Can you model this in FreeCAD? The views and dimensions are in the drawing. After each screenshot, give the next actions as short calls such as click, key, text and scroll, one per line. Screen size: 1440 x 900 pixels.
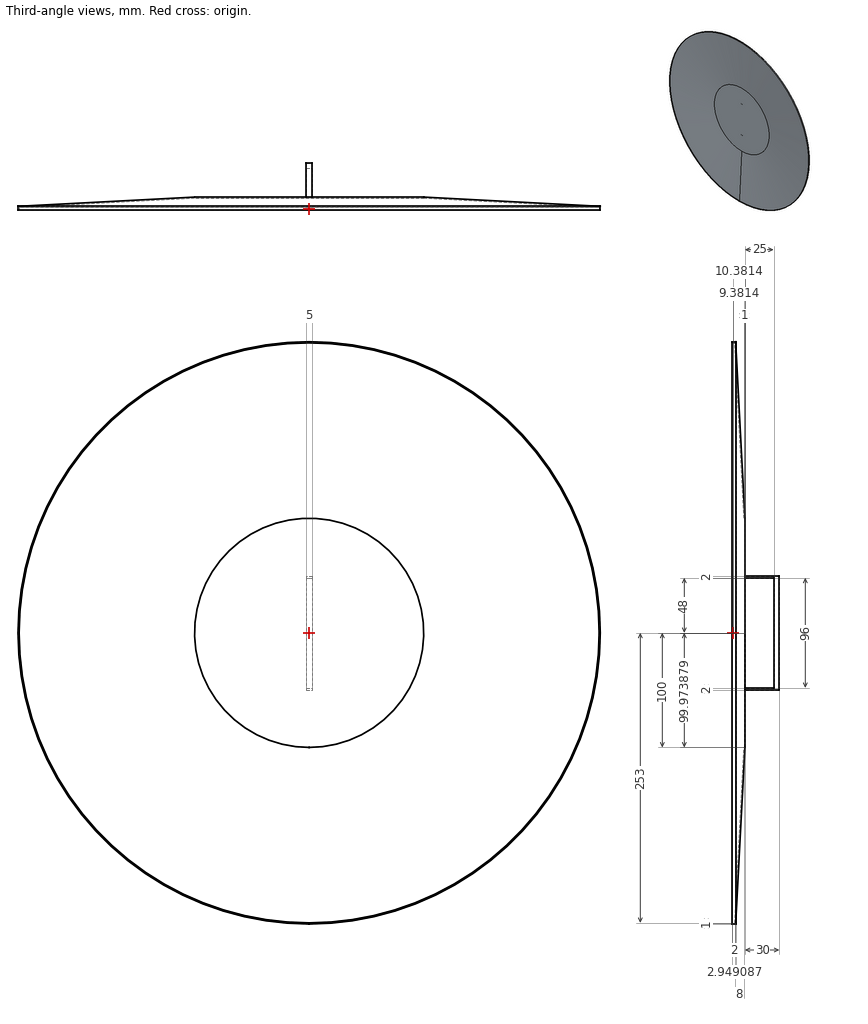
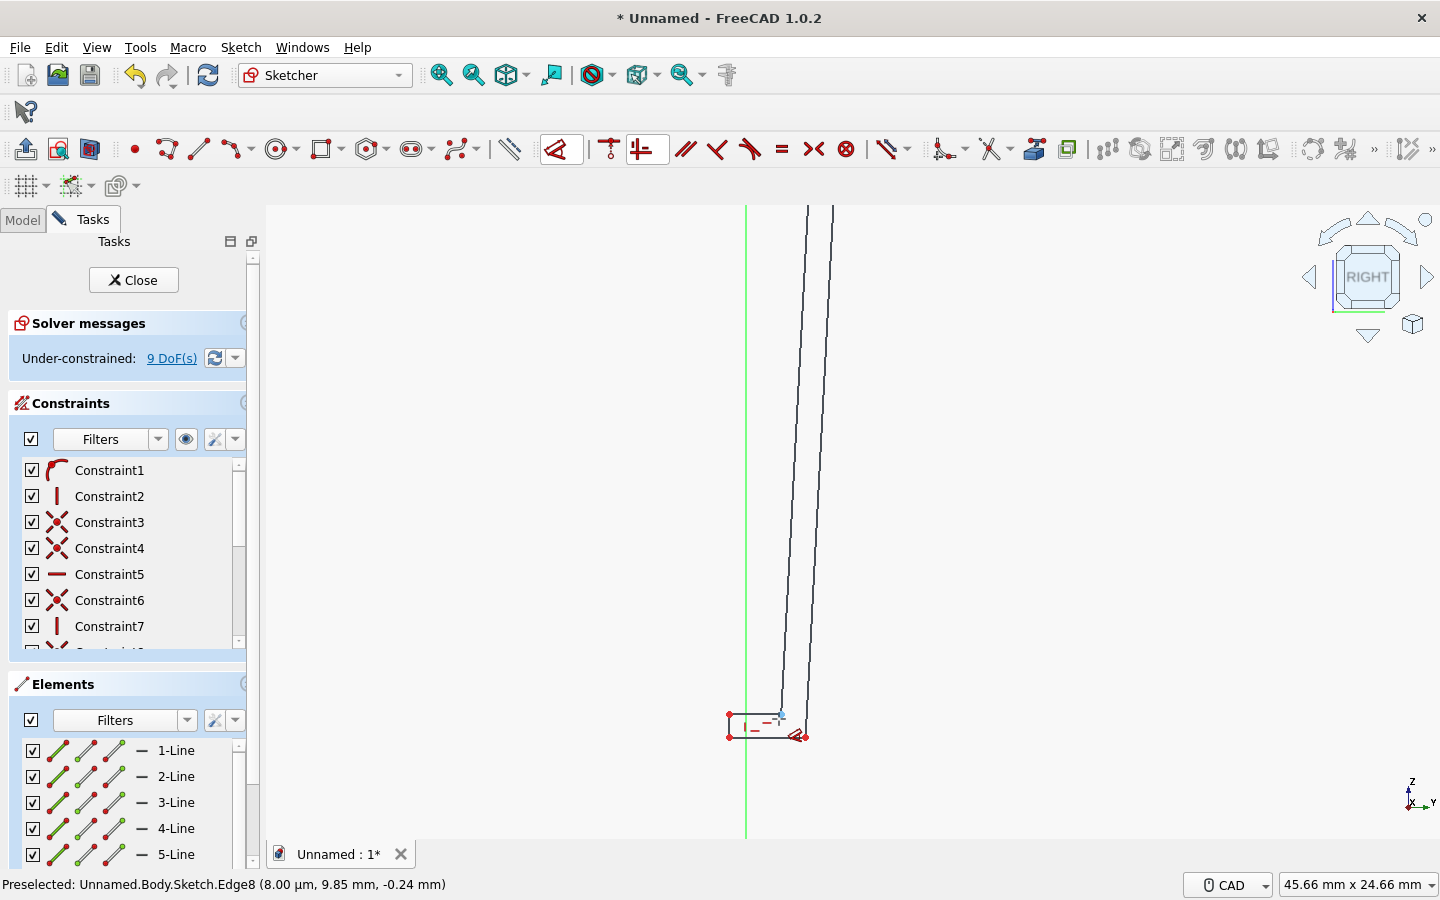
click(766, 714)
click(767, 680)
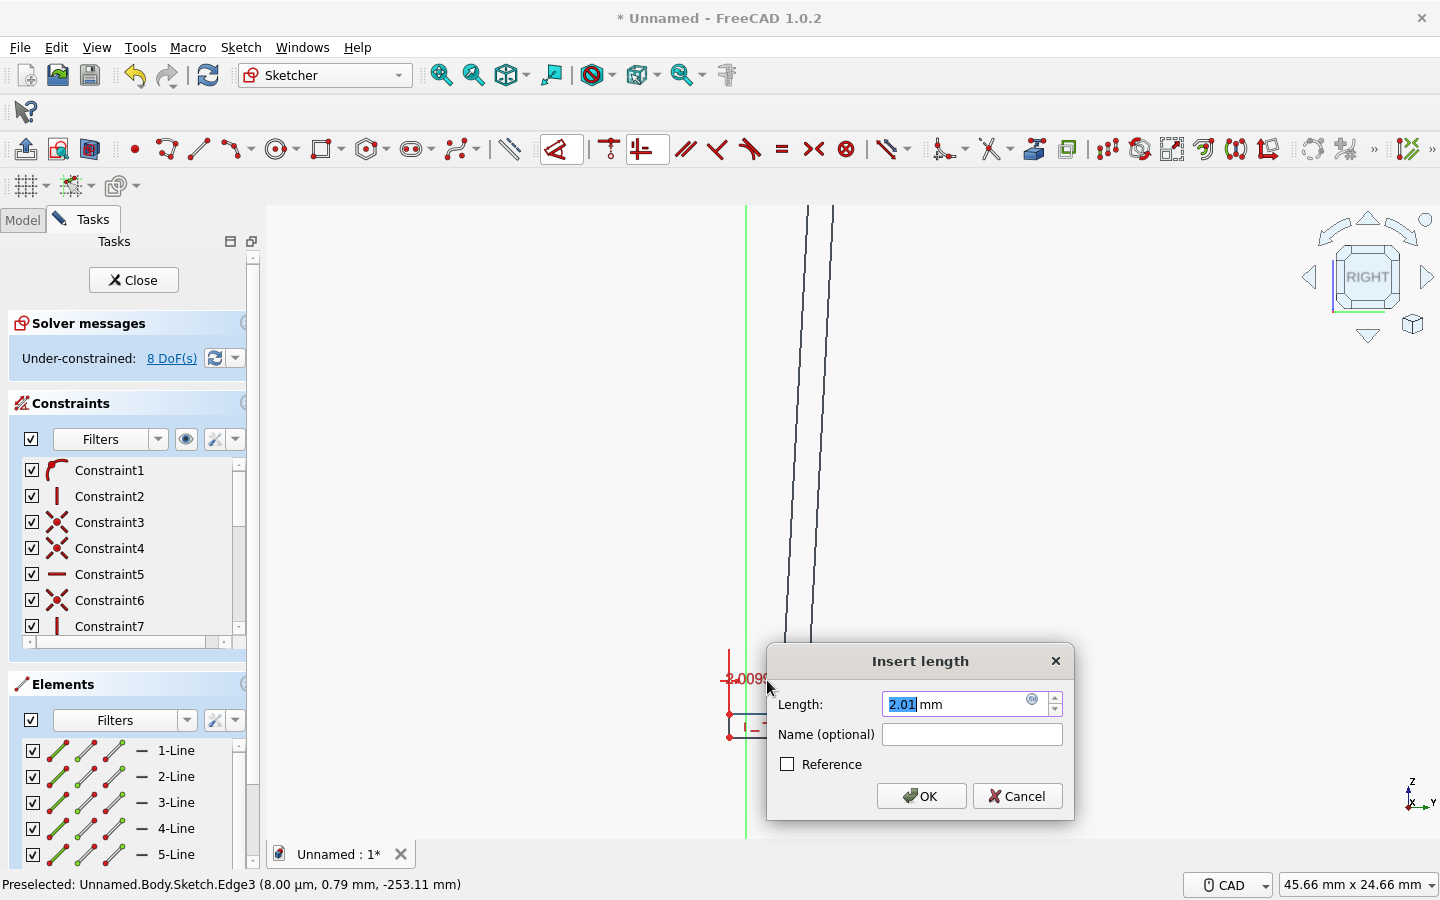
text(2)
key(Return)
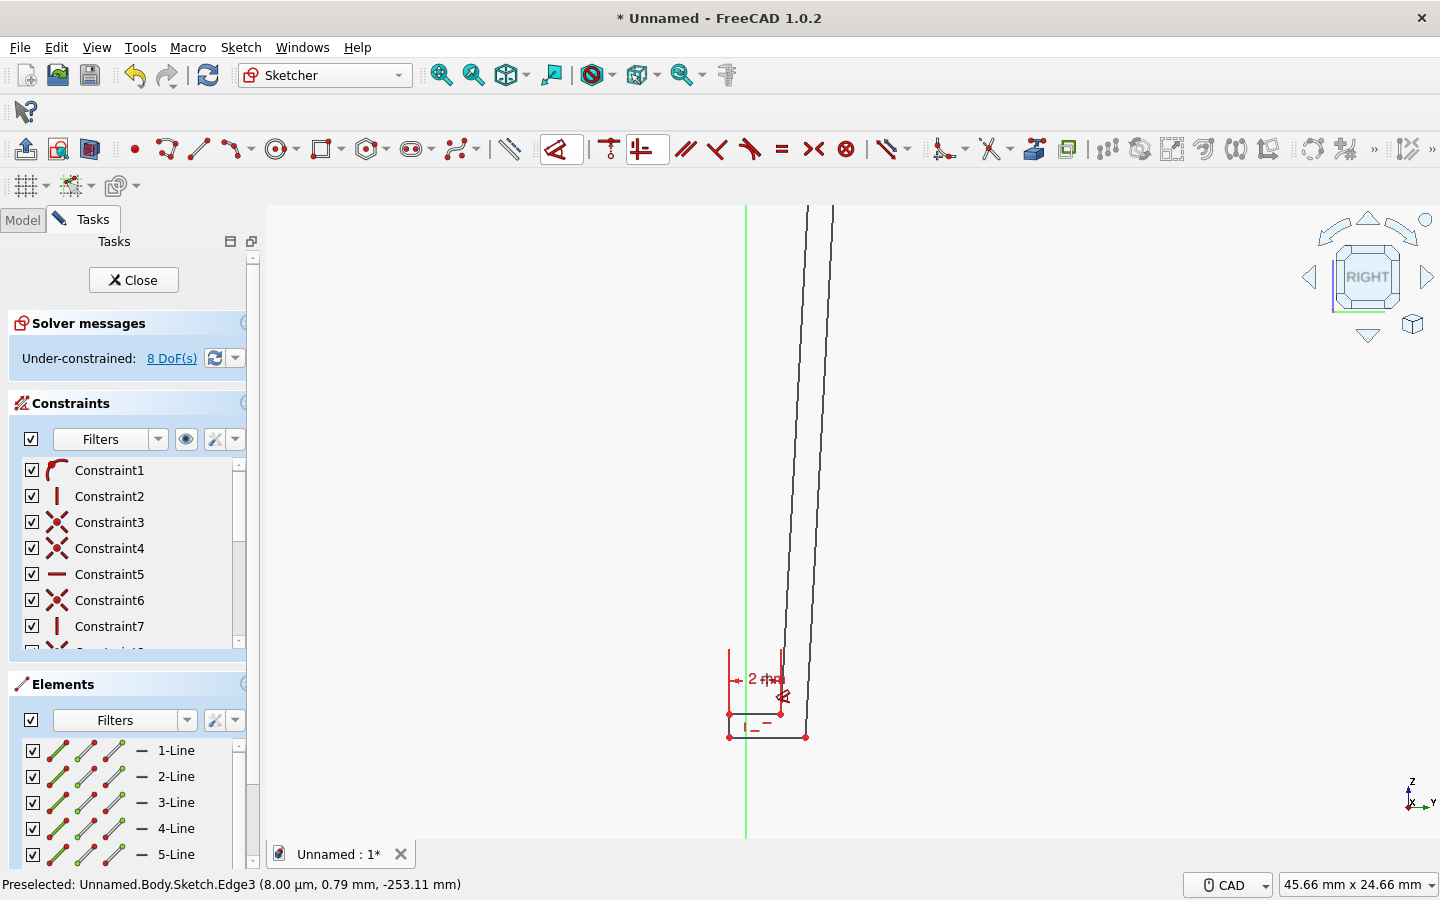
scroll(729, 724, up, 3)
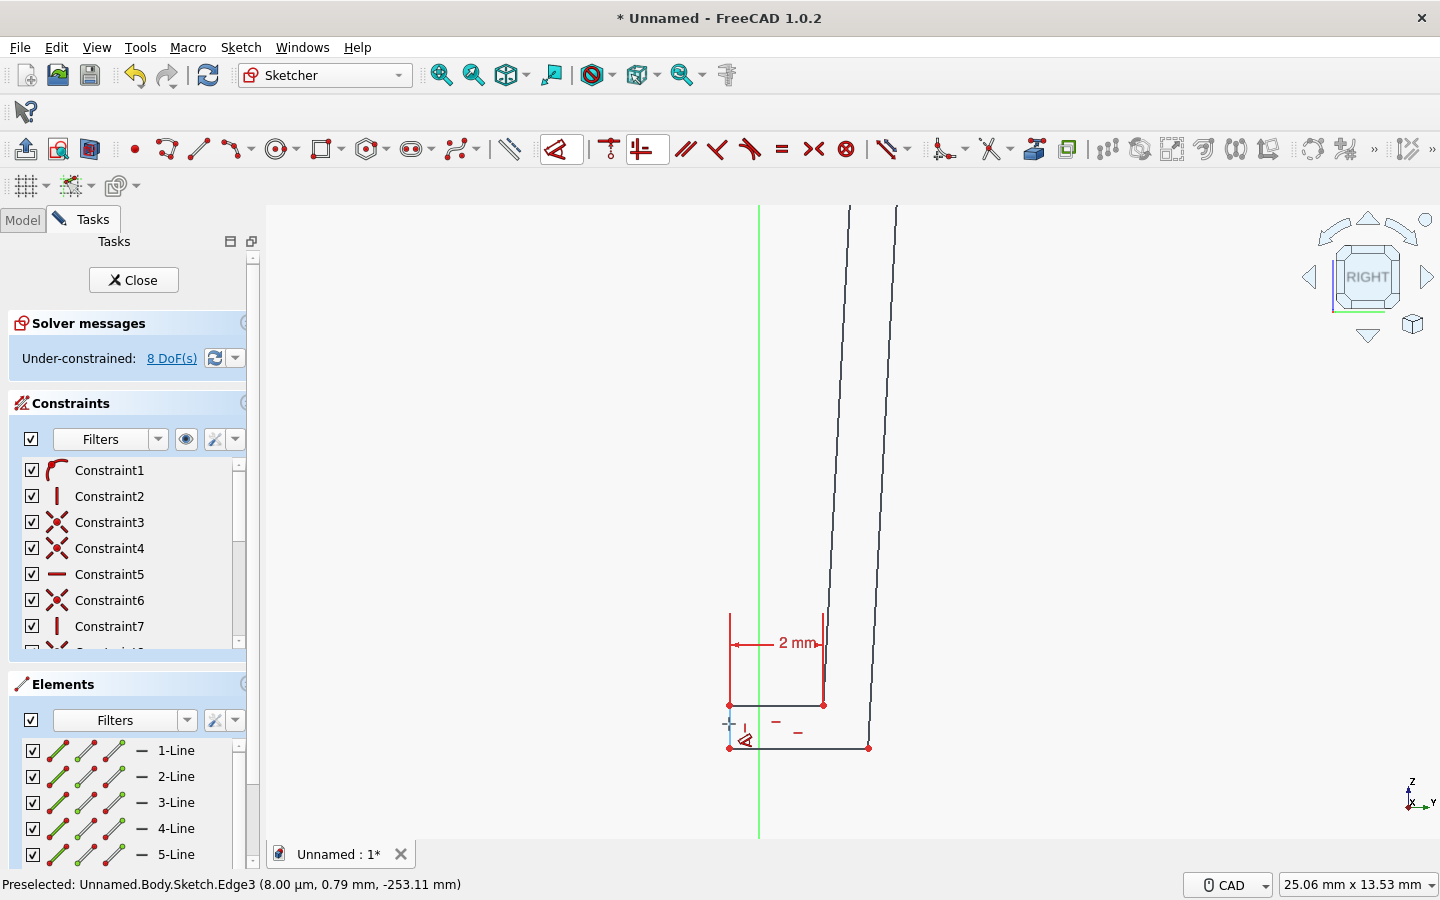
click(730, 723)
click(696, 727)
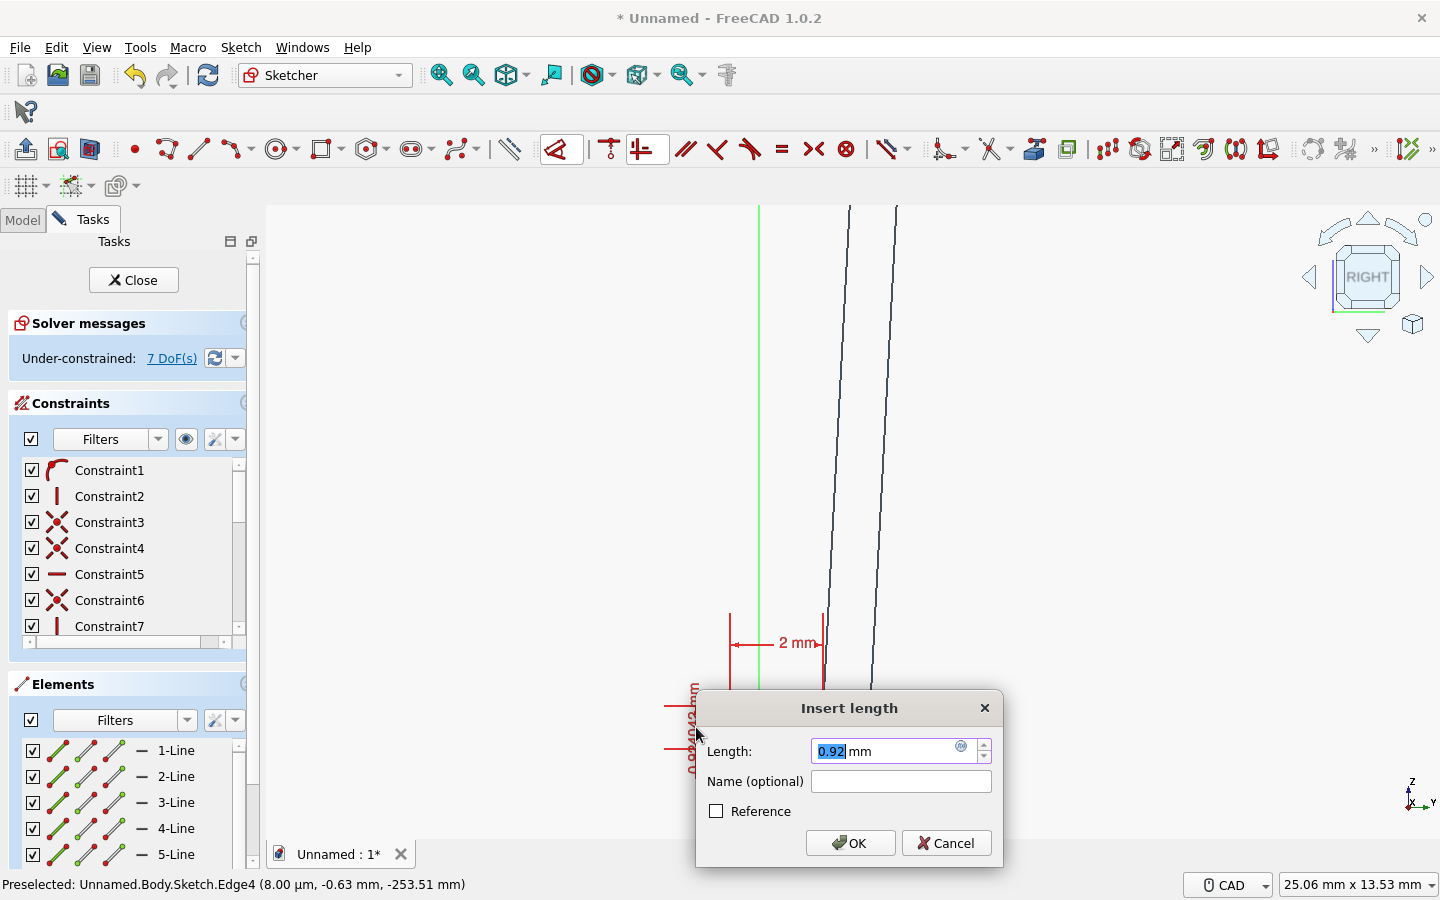
text(1)
key(Return)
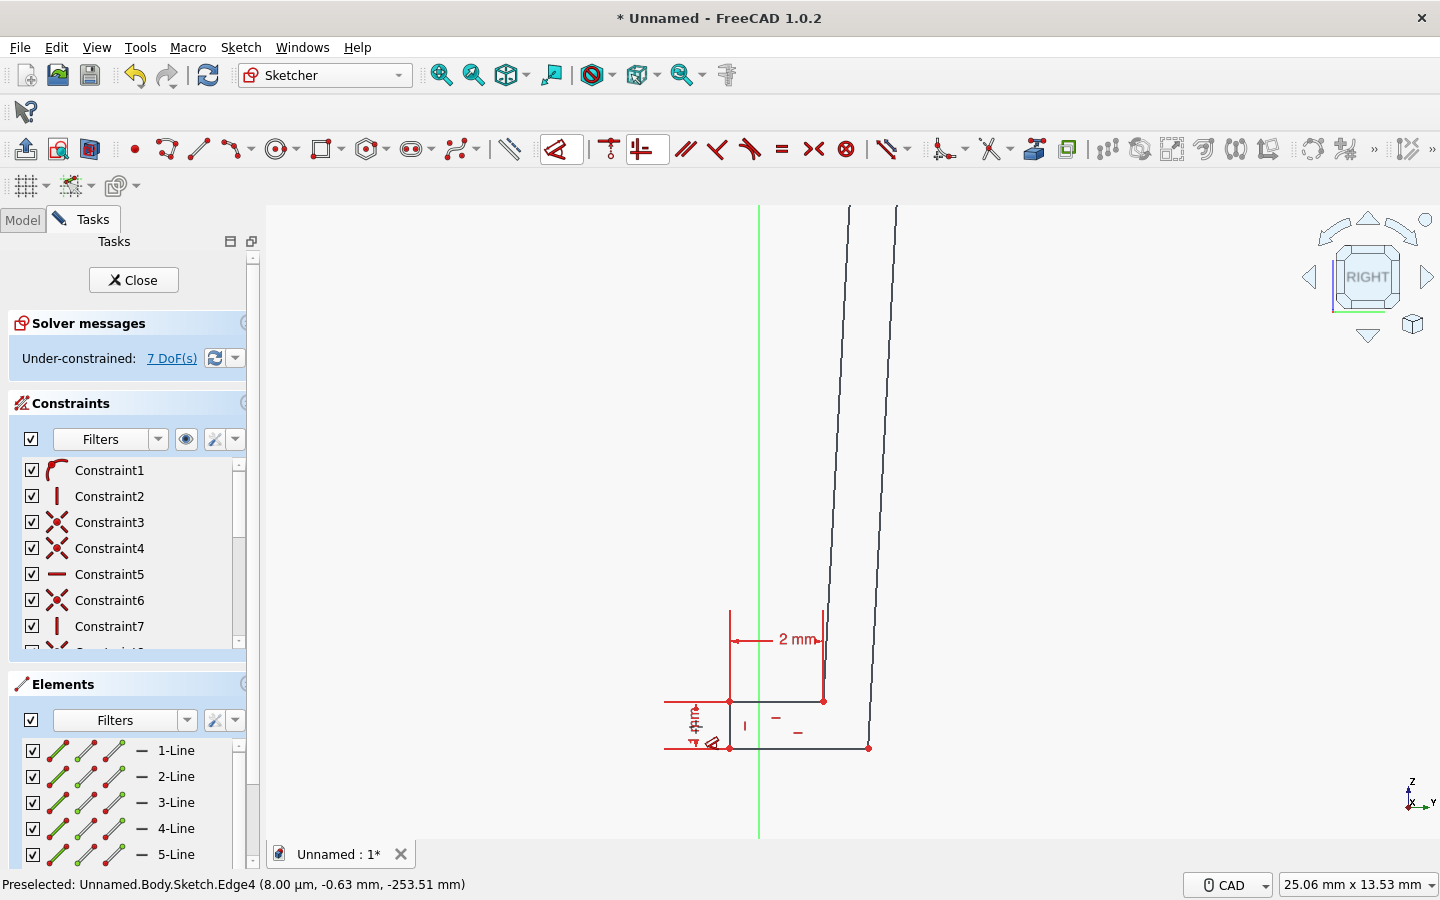
scroll(776, 765, down, 16)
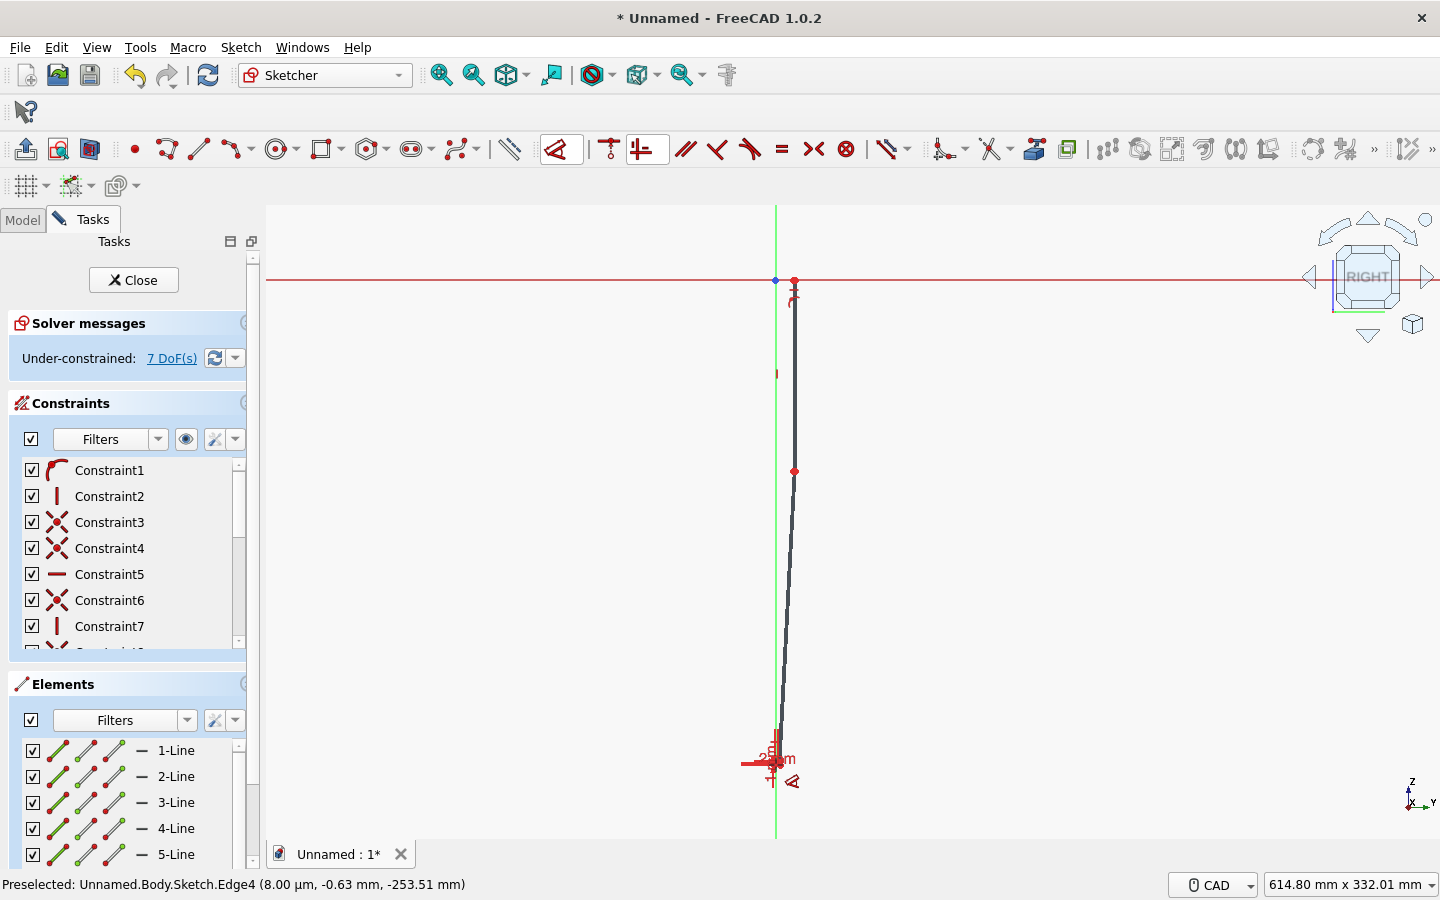
scroll(795, 280, up, 16)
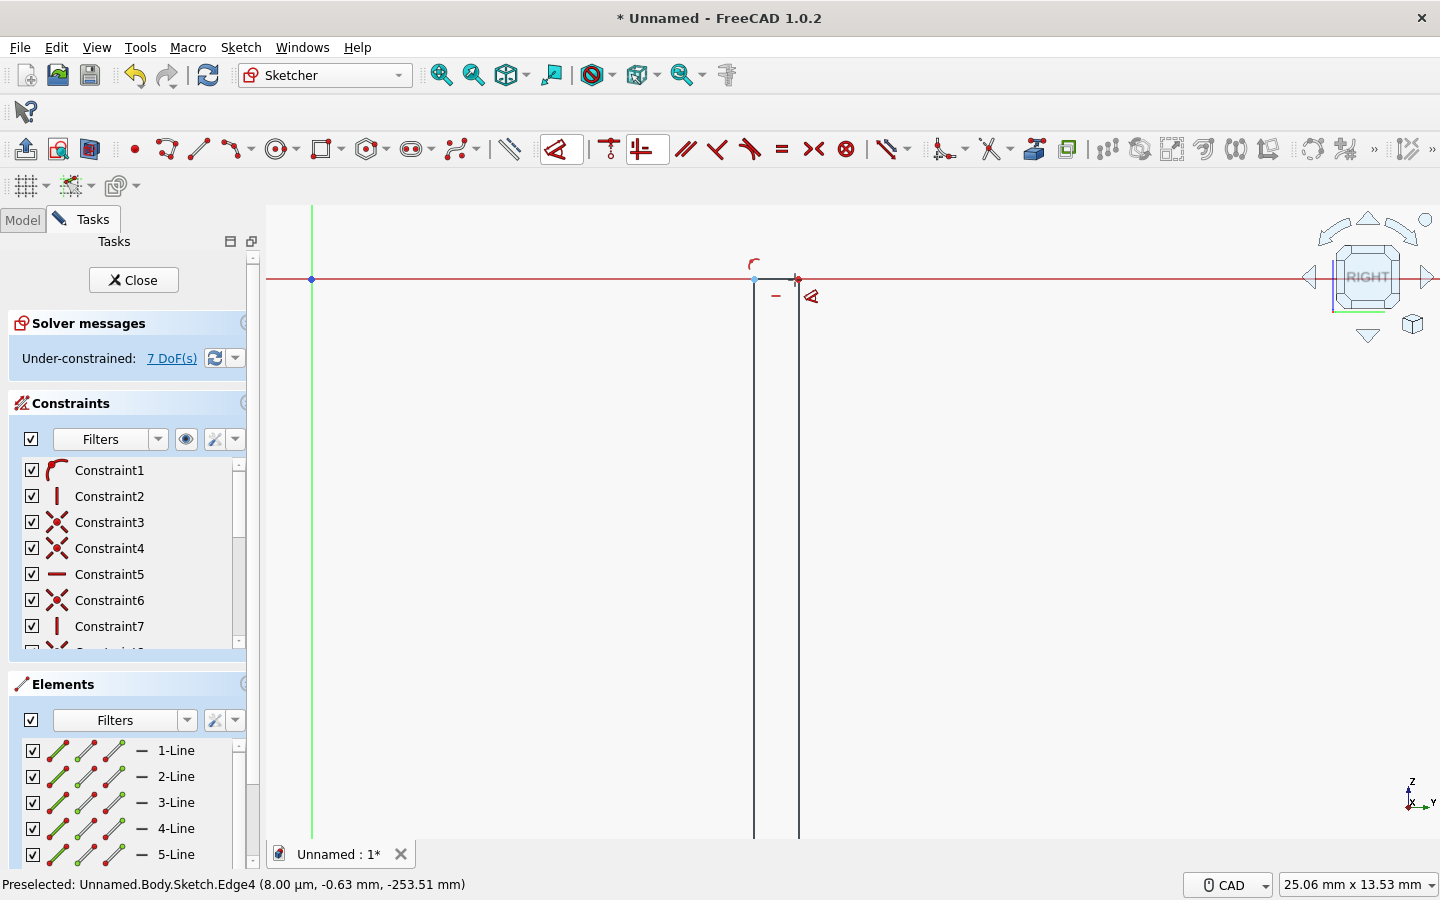
click(786, 279)
click(777, 245)